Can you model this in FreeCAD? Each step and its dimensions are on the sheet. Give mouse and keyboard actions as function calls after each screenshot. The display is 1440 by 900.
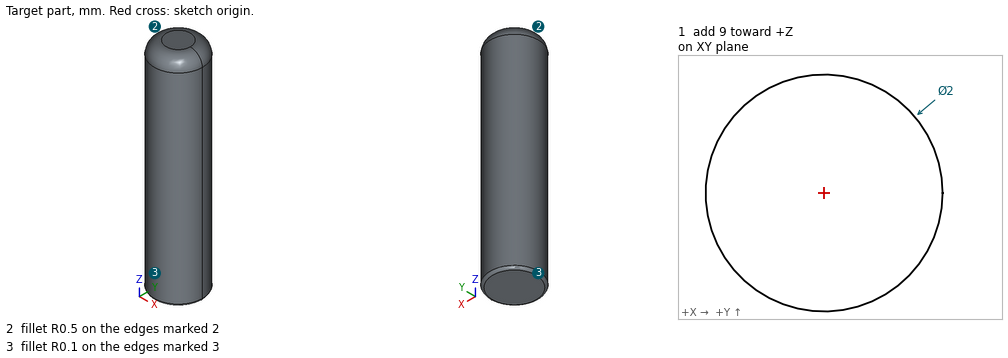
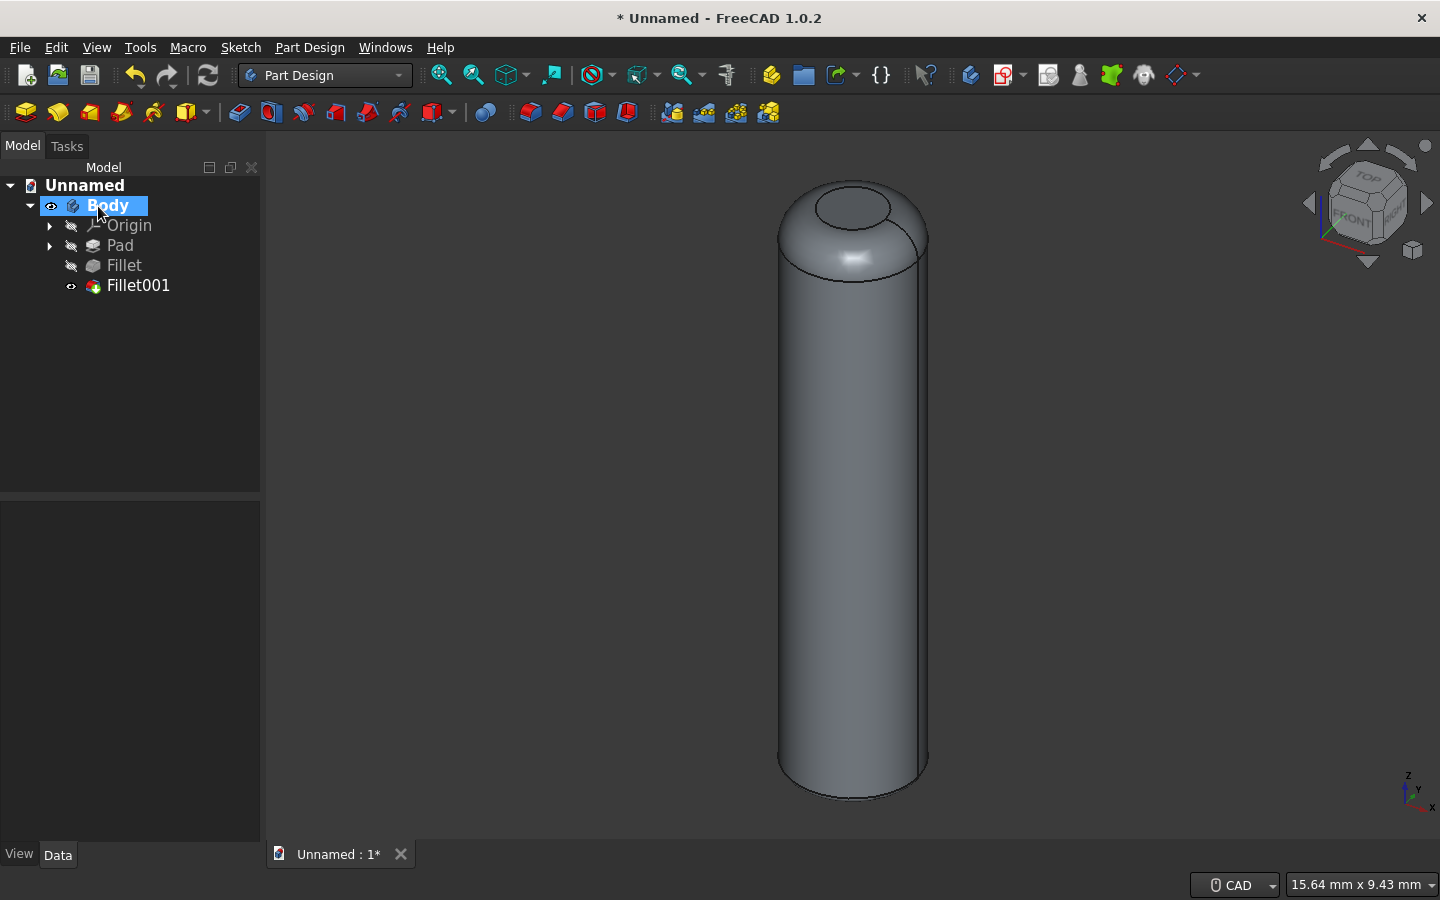
key(0)